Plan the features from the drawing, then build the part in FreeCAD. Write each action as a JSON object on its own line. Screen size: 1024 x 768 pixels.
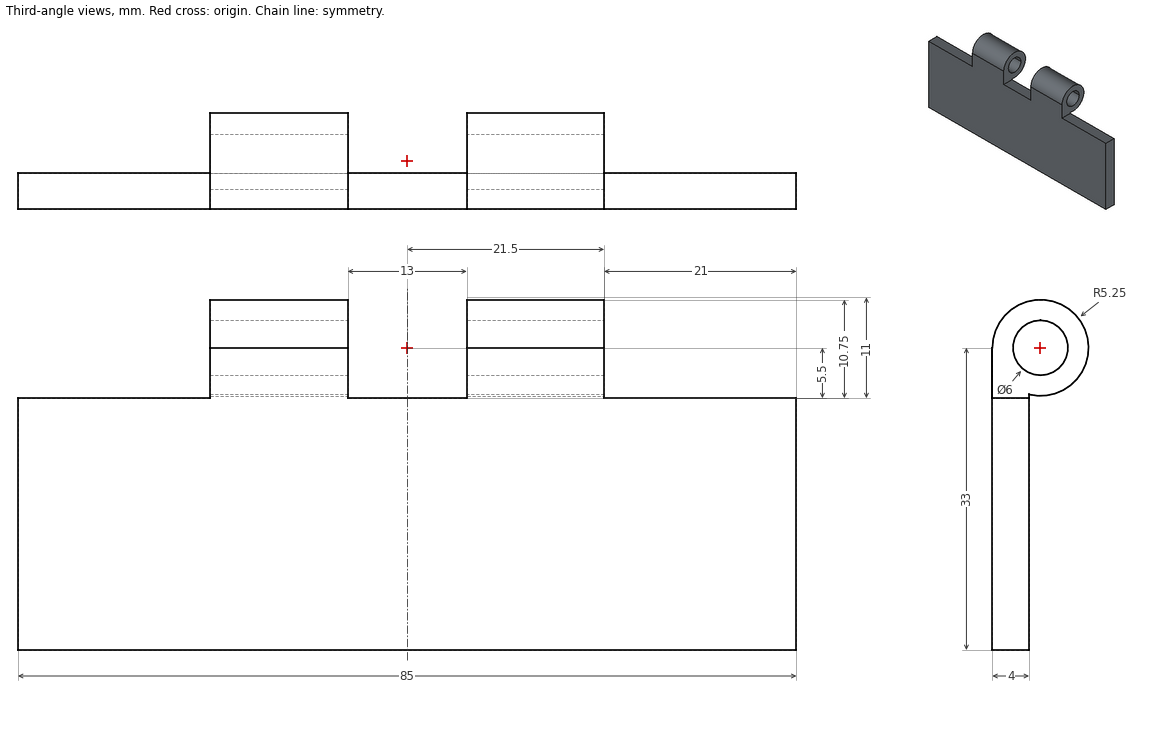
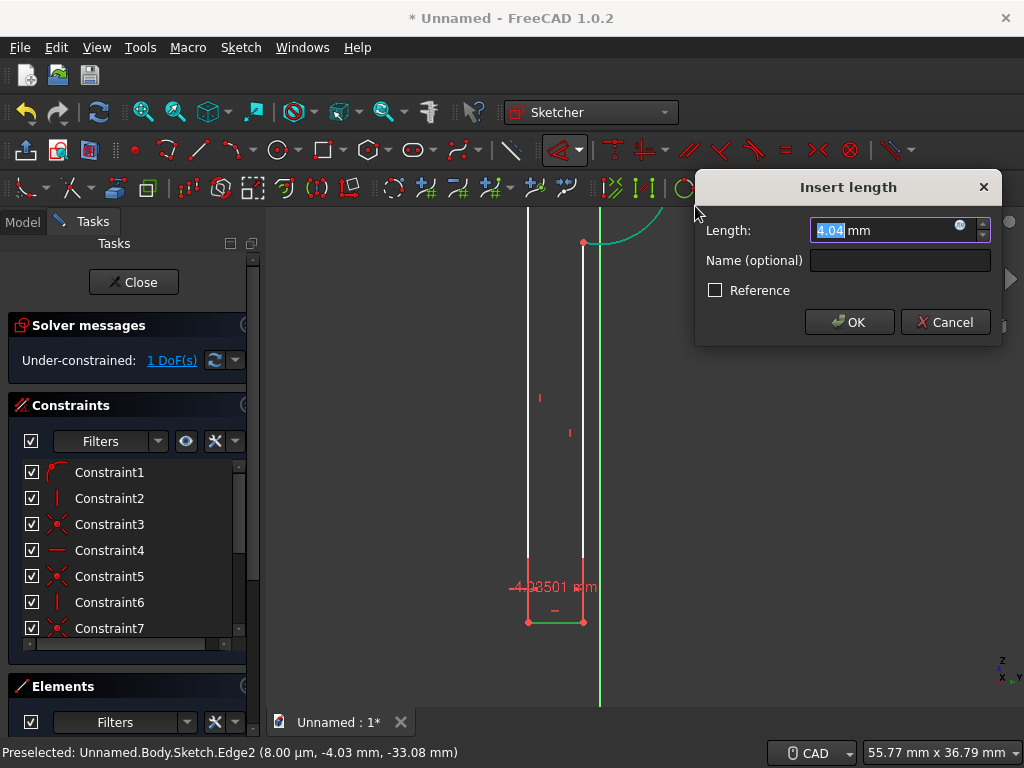
{"action": "type", "text": "4"}
{"action": "key", "text": "Return"}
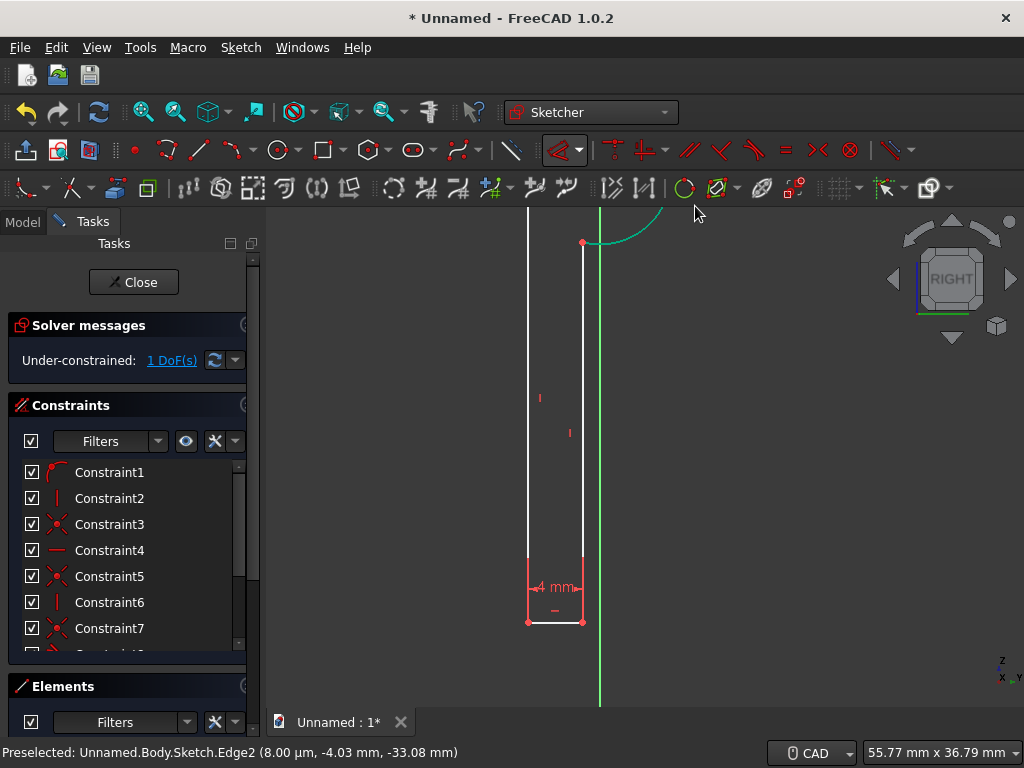
{"action": "left_click", "coordinate": [528, 308]}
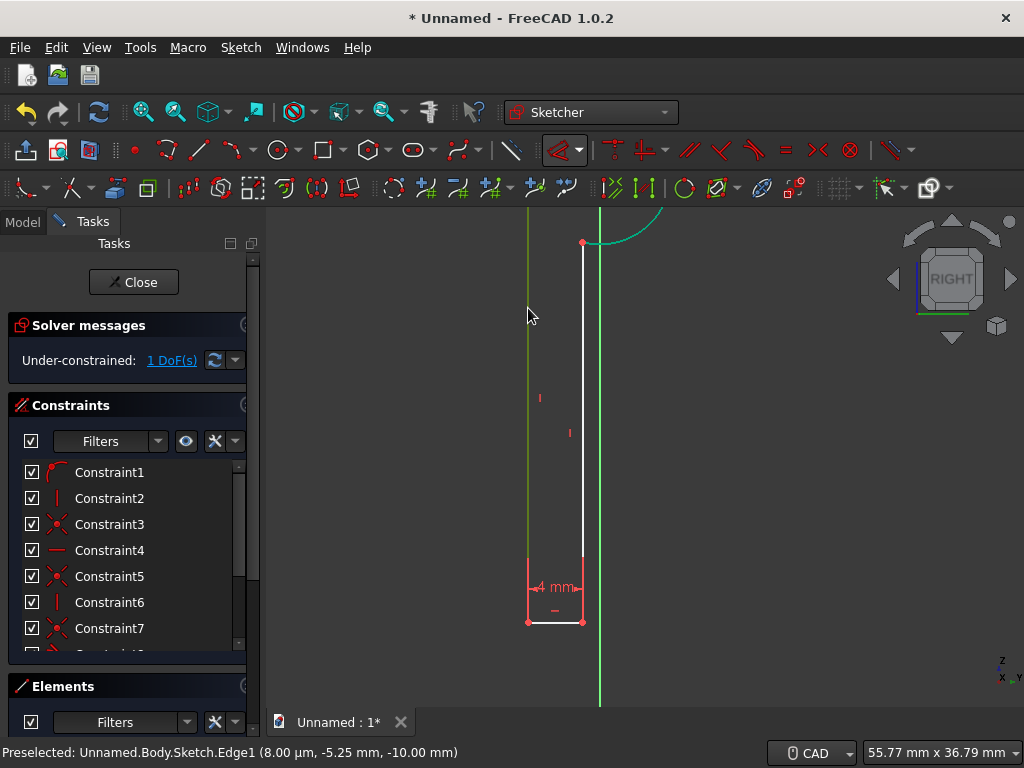
{"action": "key", "text": "i"}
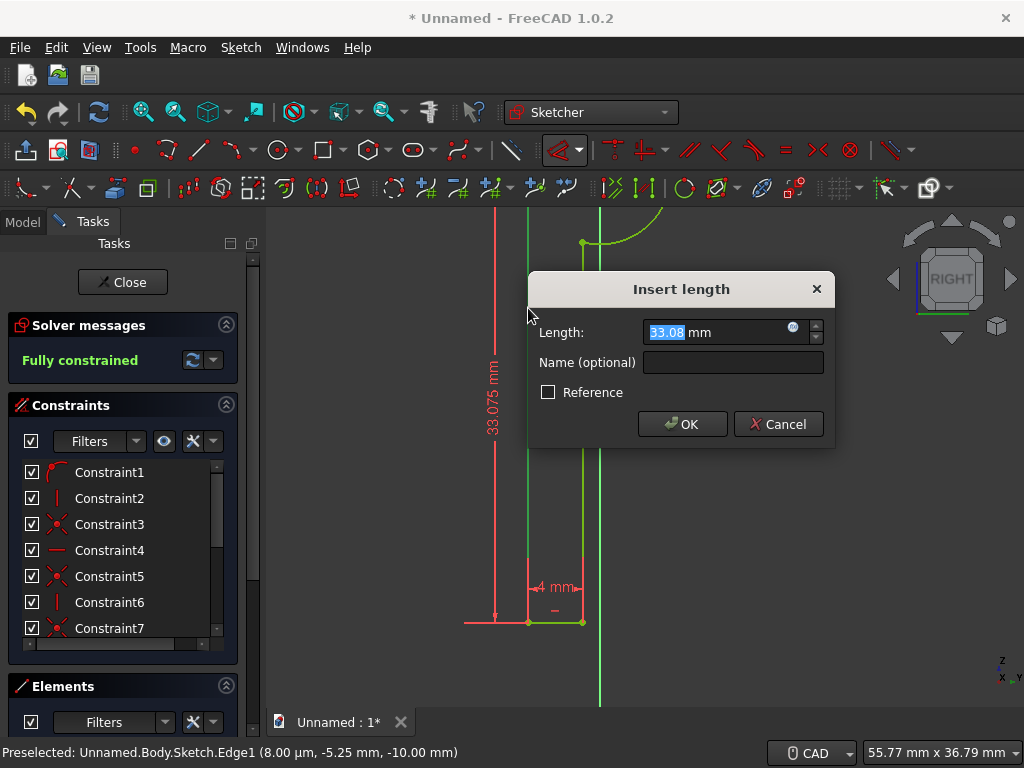
{"action": "type", "text": "33"}
{"action": "key", "text": "Return"}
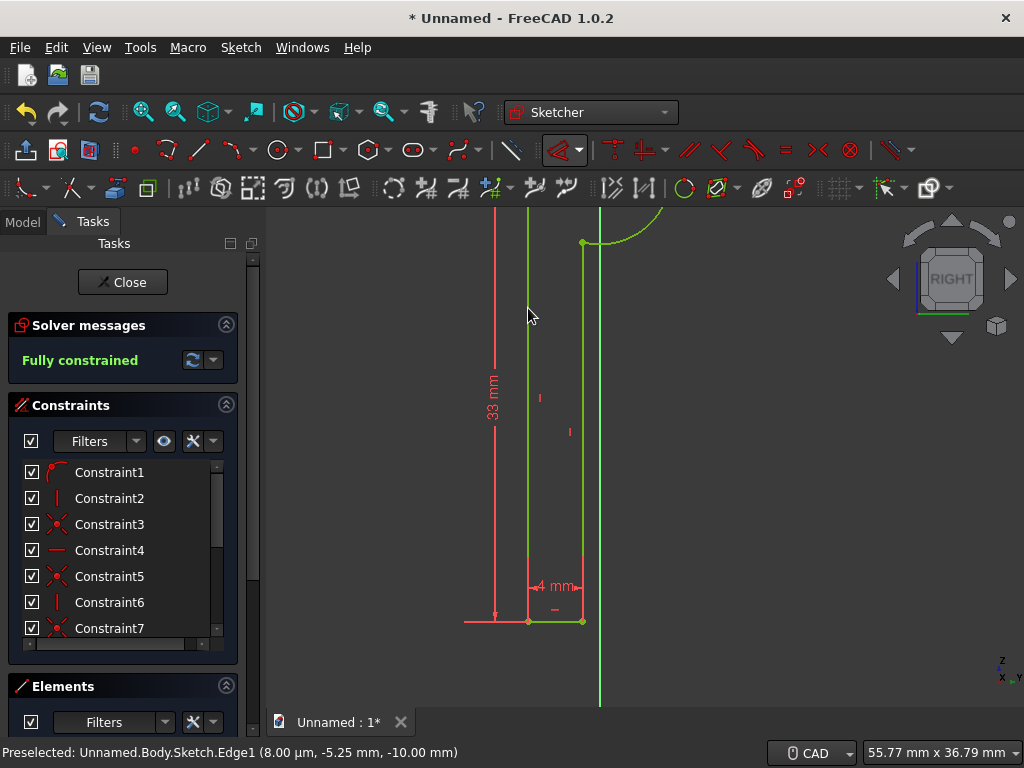
{"action": "left_click", "coordinate": [123, 282]}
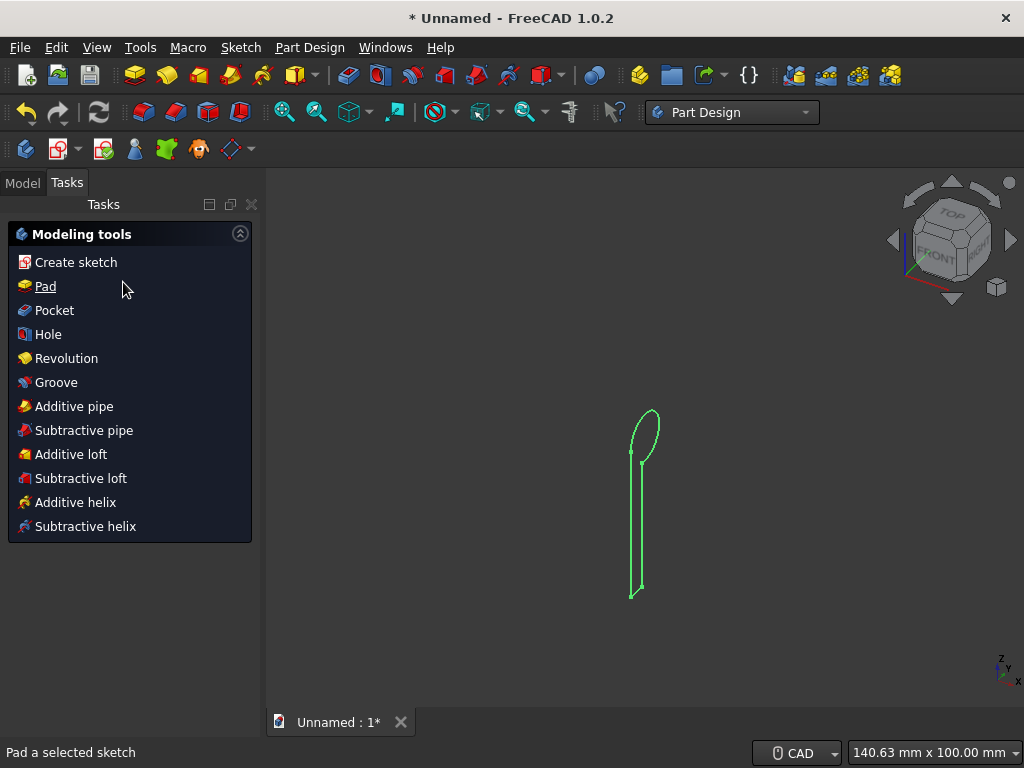
{"action": "left_click", "coordinate": [136, 76]}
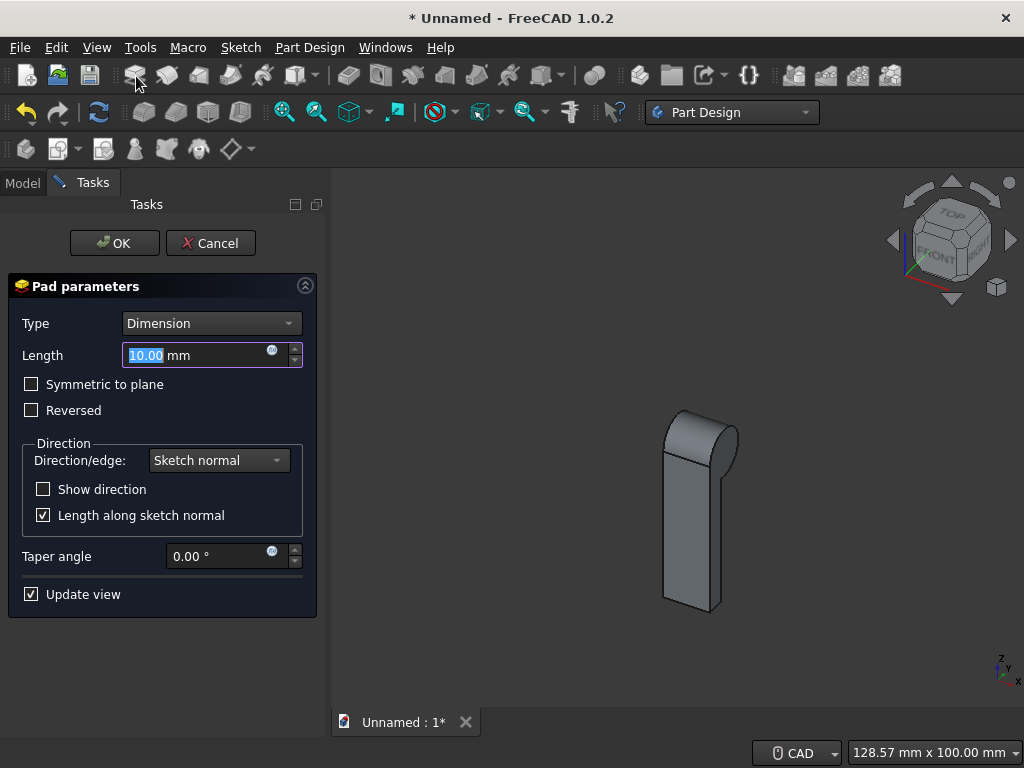
{"action": "type", "text": "85"}
{"action": "key", "text": "Tab"}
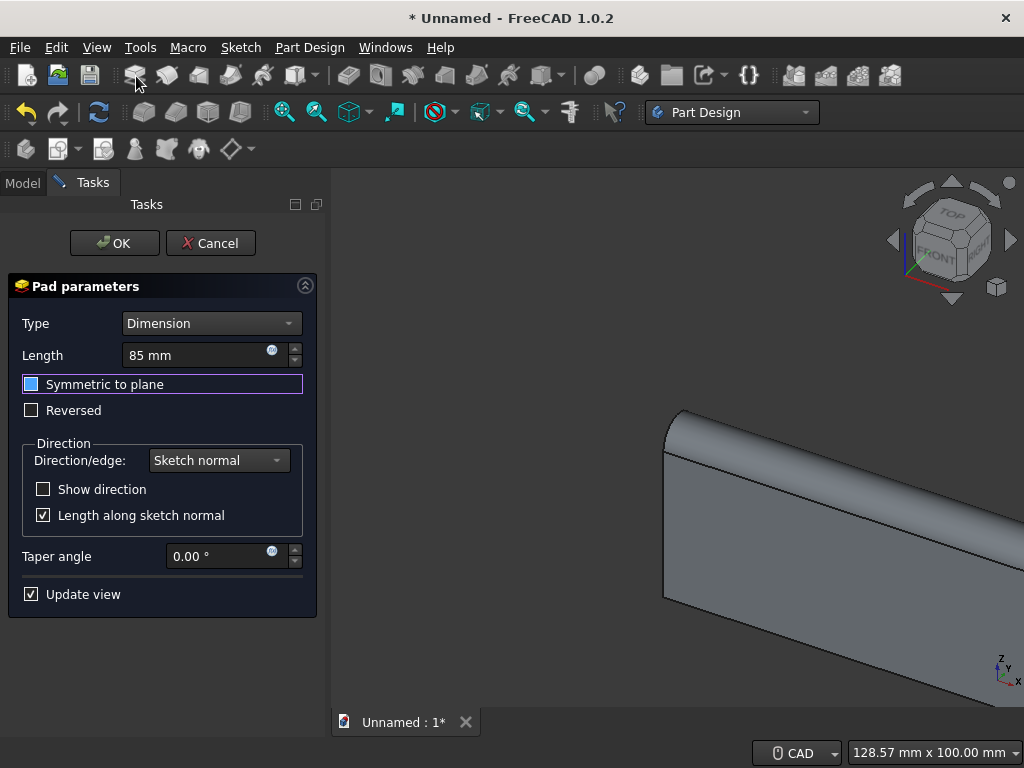
{"action": "left_click", "coordinate": [30, 384]}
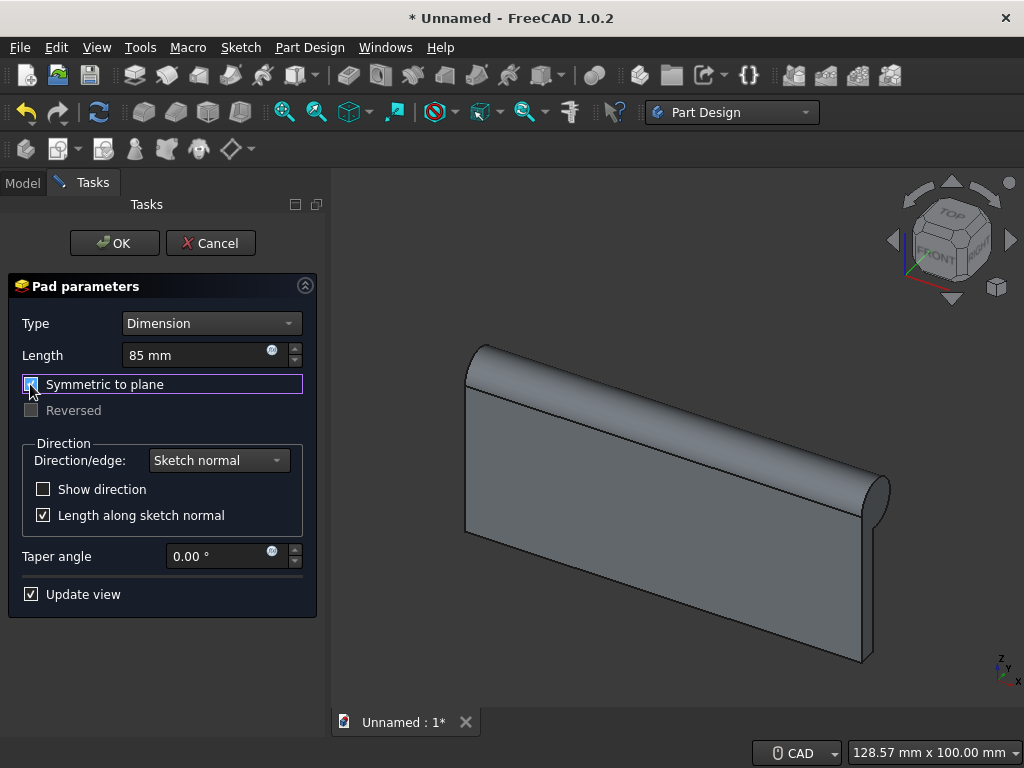
{"action": "left_click", "coordinate": [115, 243]}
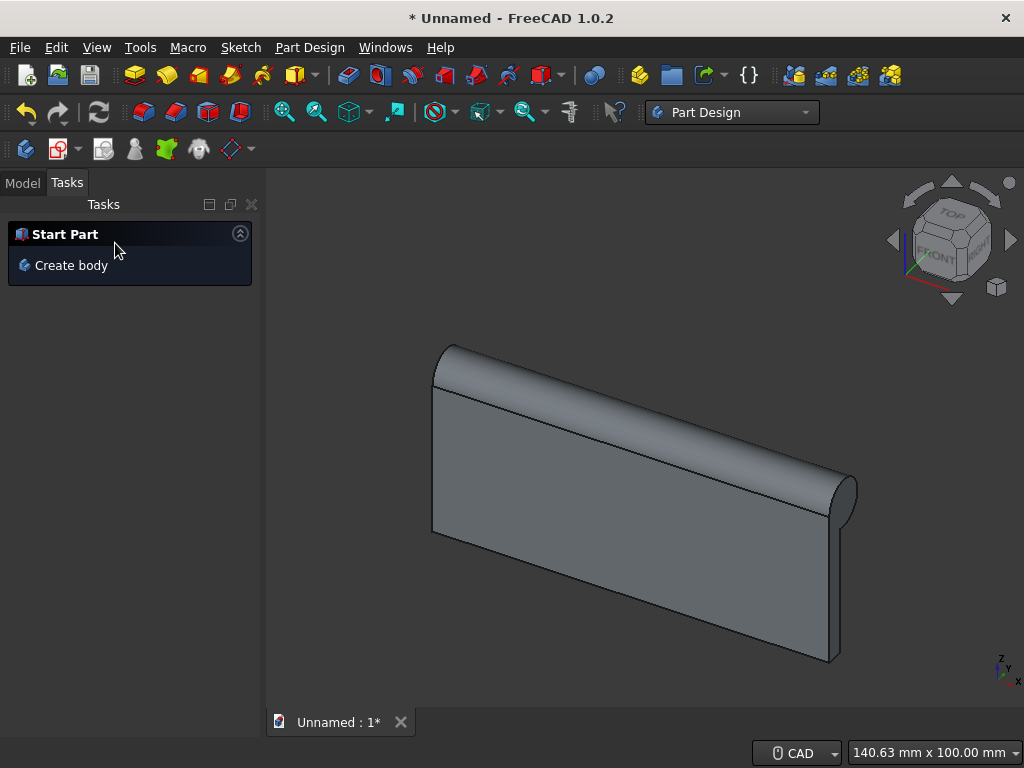
{"action": "left_click", "coordinate": [58, 150]}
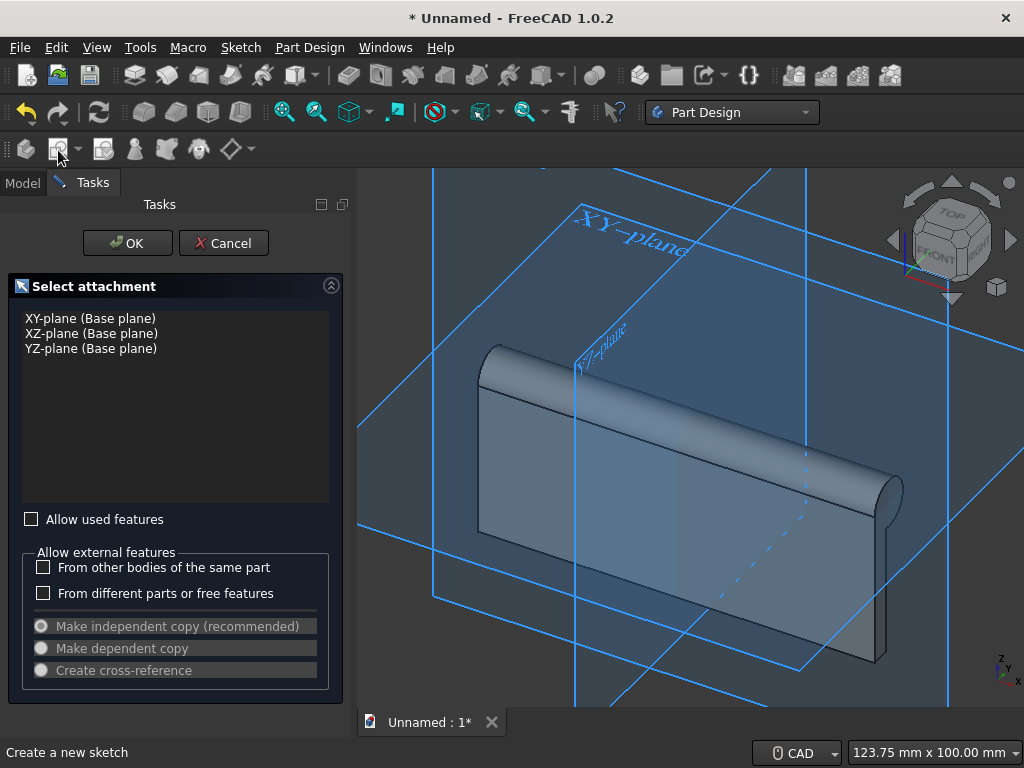
{"action": "left_click", "coordinate": [82, 334]}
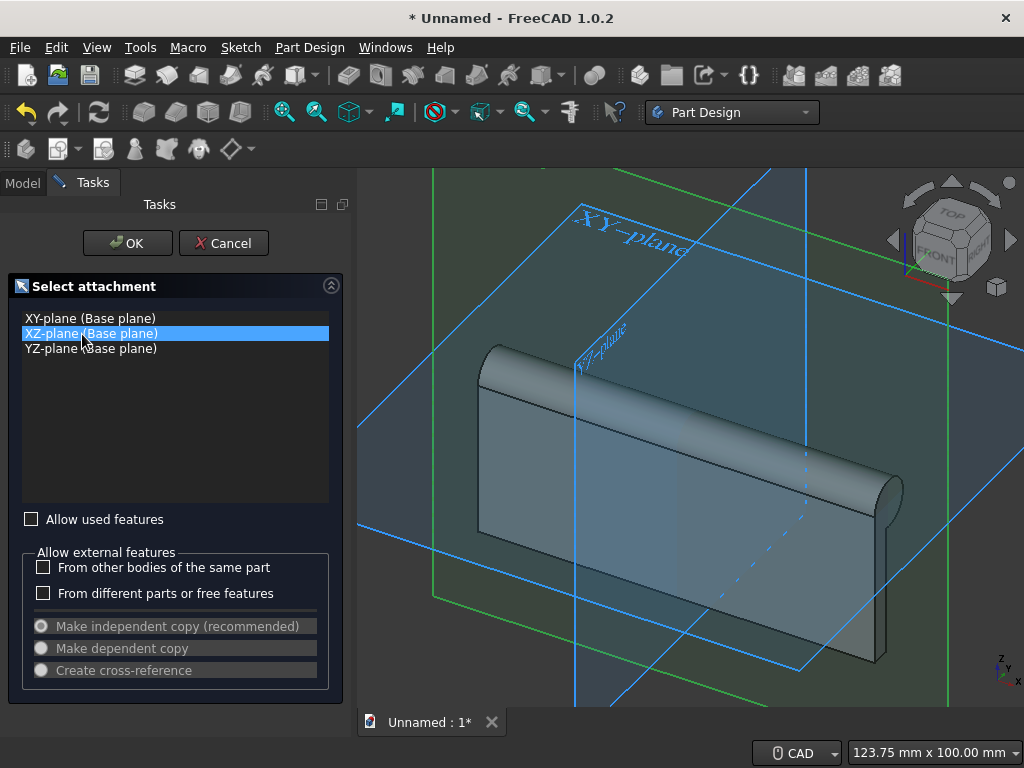
{"action": "left_click", "coordinate": [128, 243]}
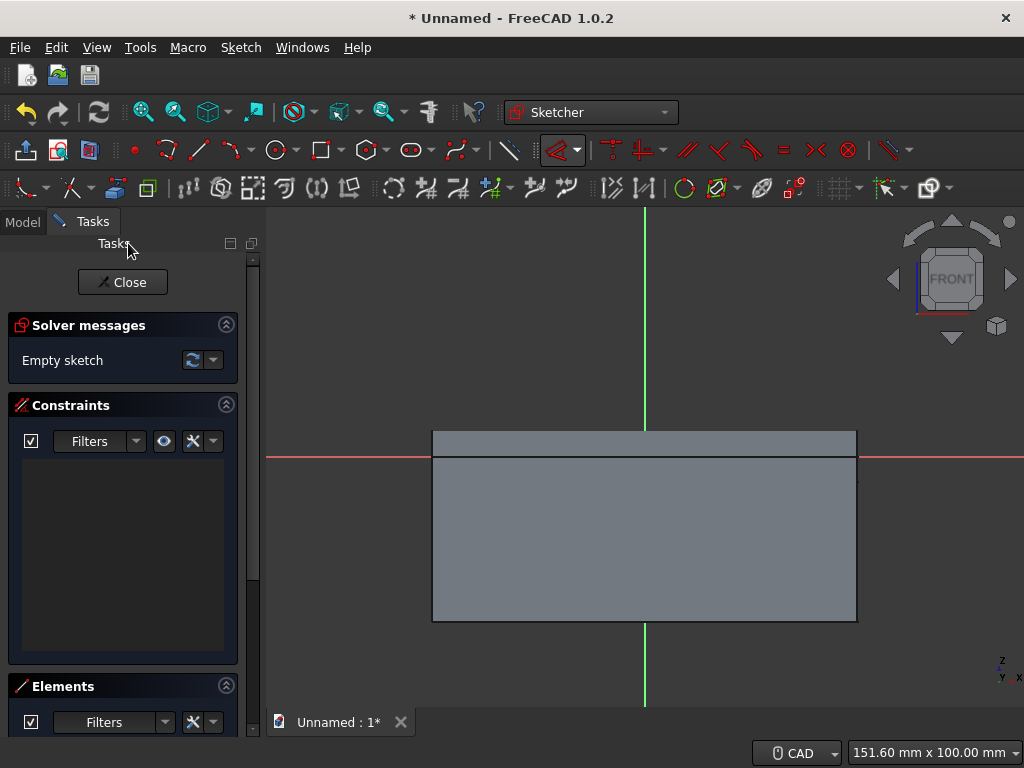
{"action": "left_click", "coordinate": [90, 150]}